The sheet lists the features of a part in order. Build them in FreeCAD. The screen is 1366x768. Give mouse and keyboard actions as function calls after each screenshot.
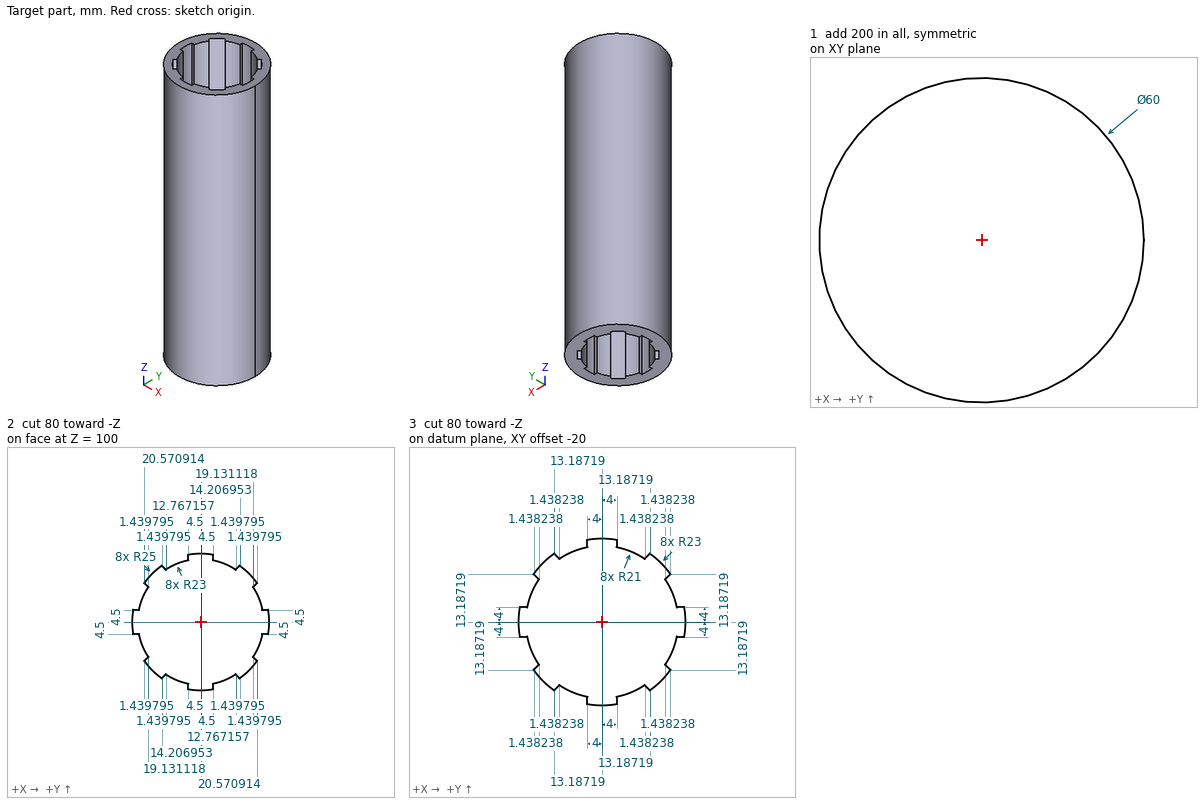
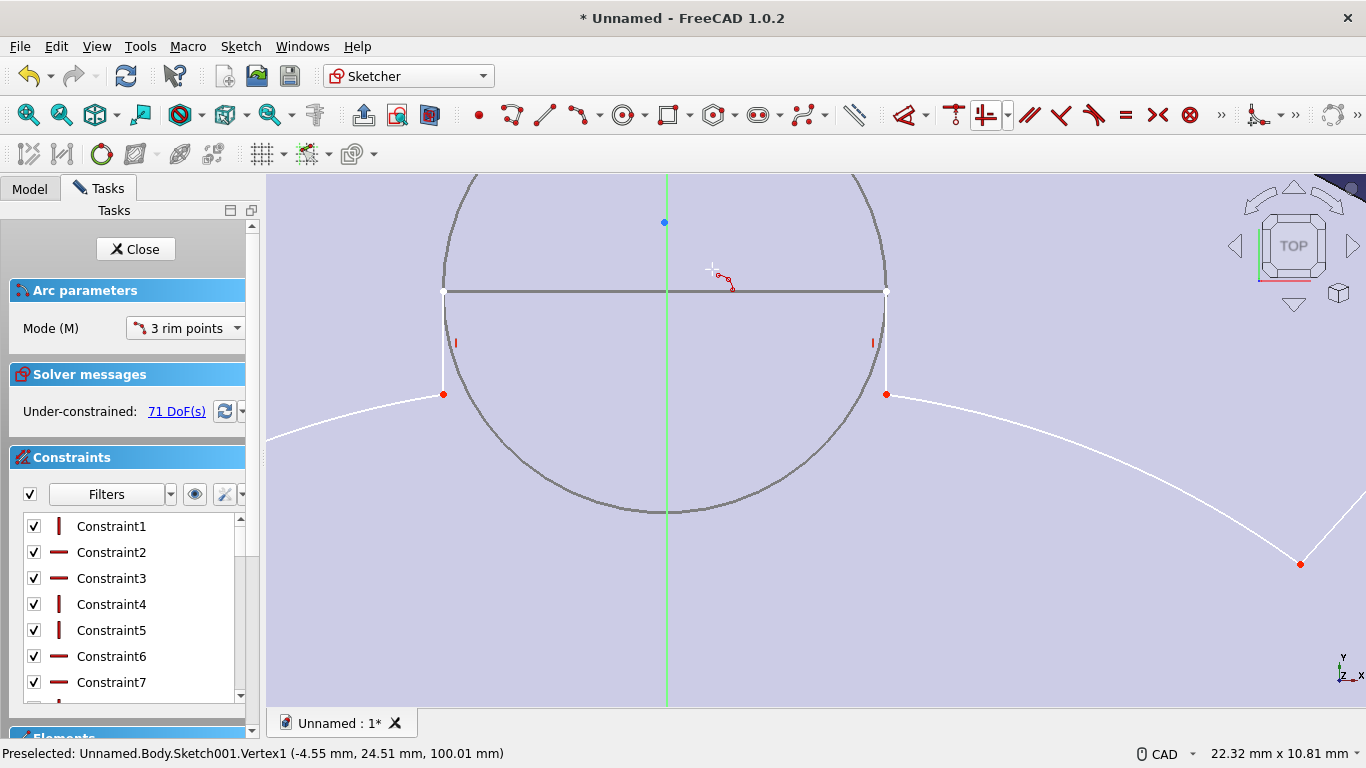
click(712, 268)
key(Escape)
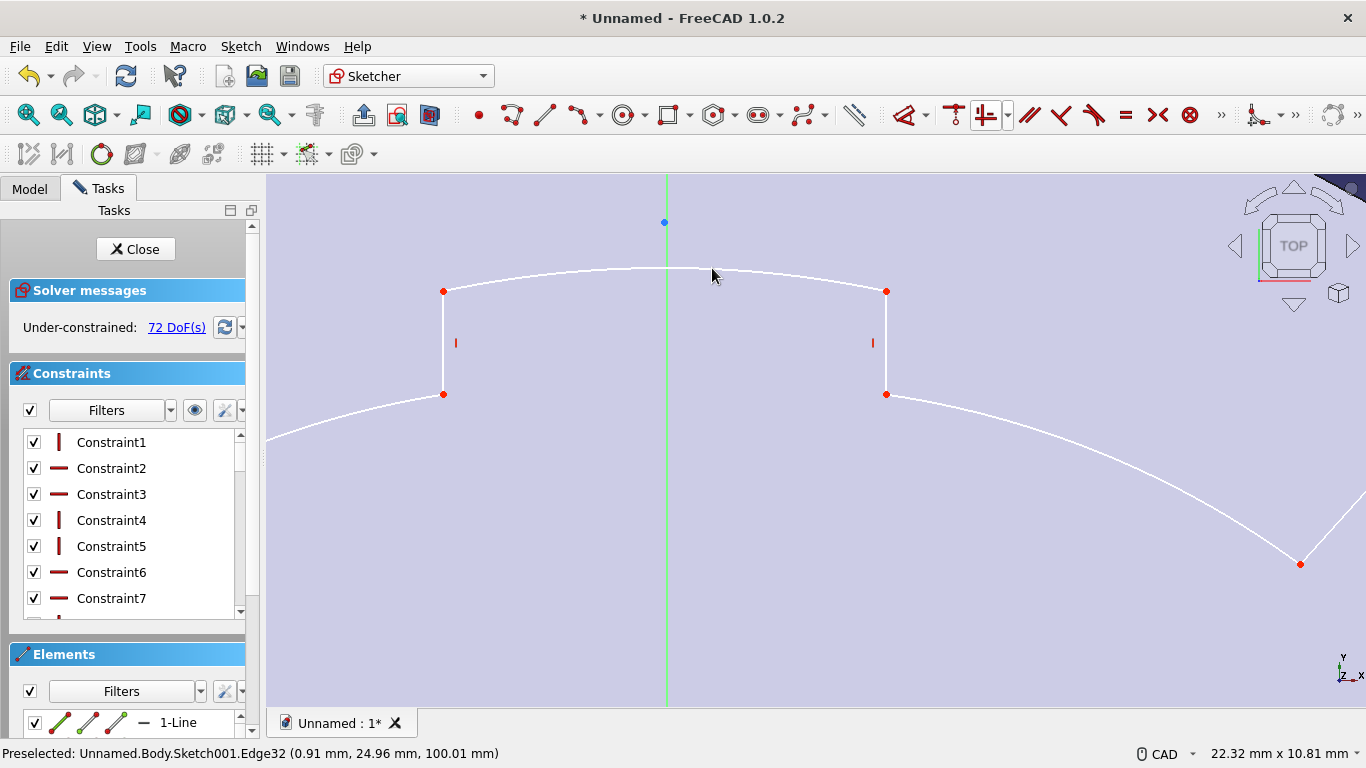
scroll(760, 275, down, 10)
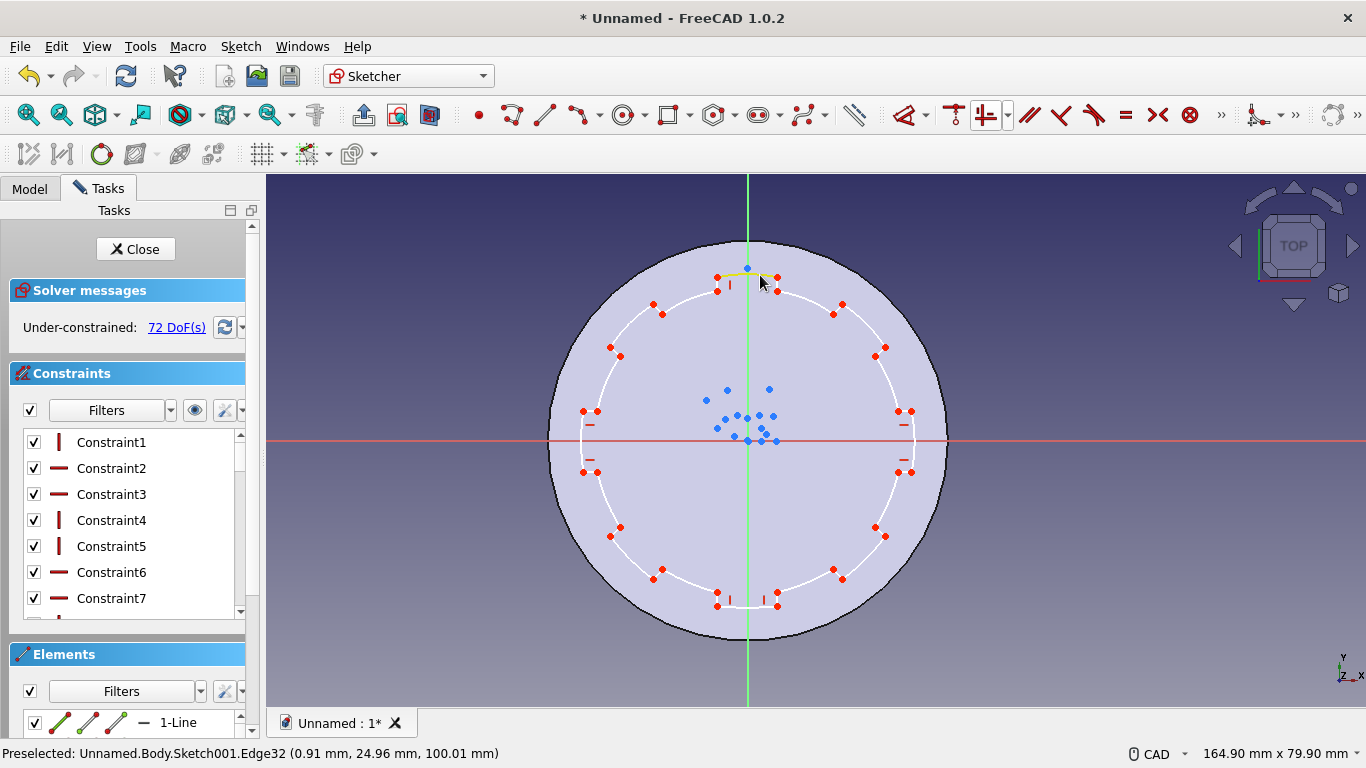
click(700, 295)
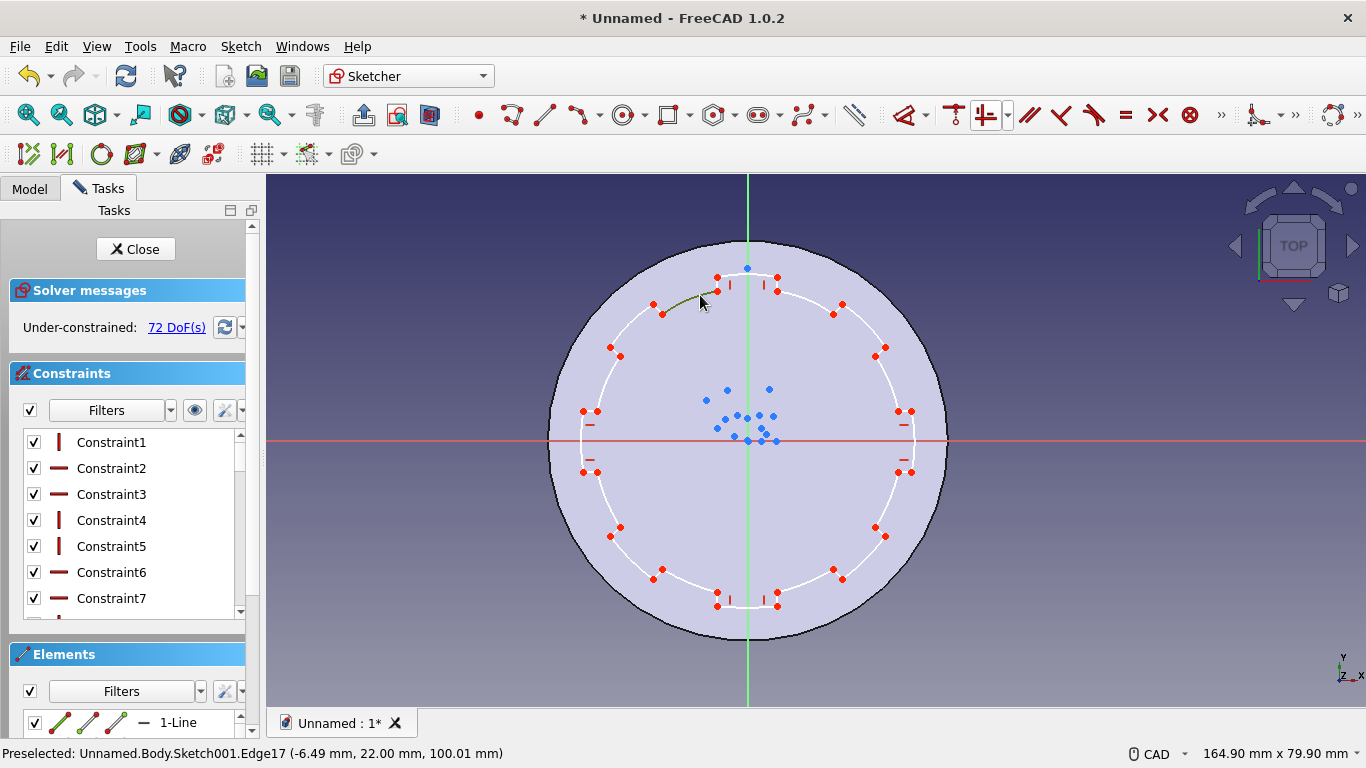
click(639, 315)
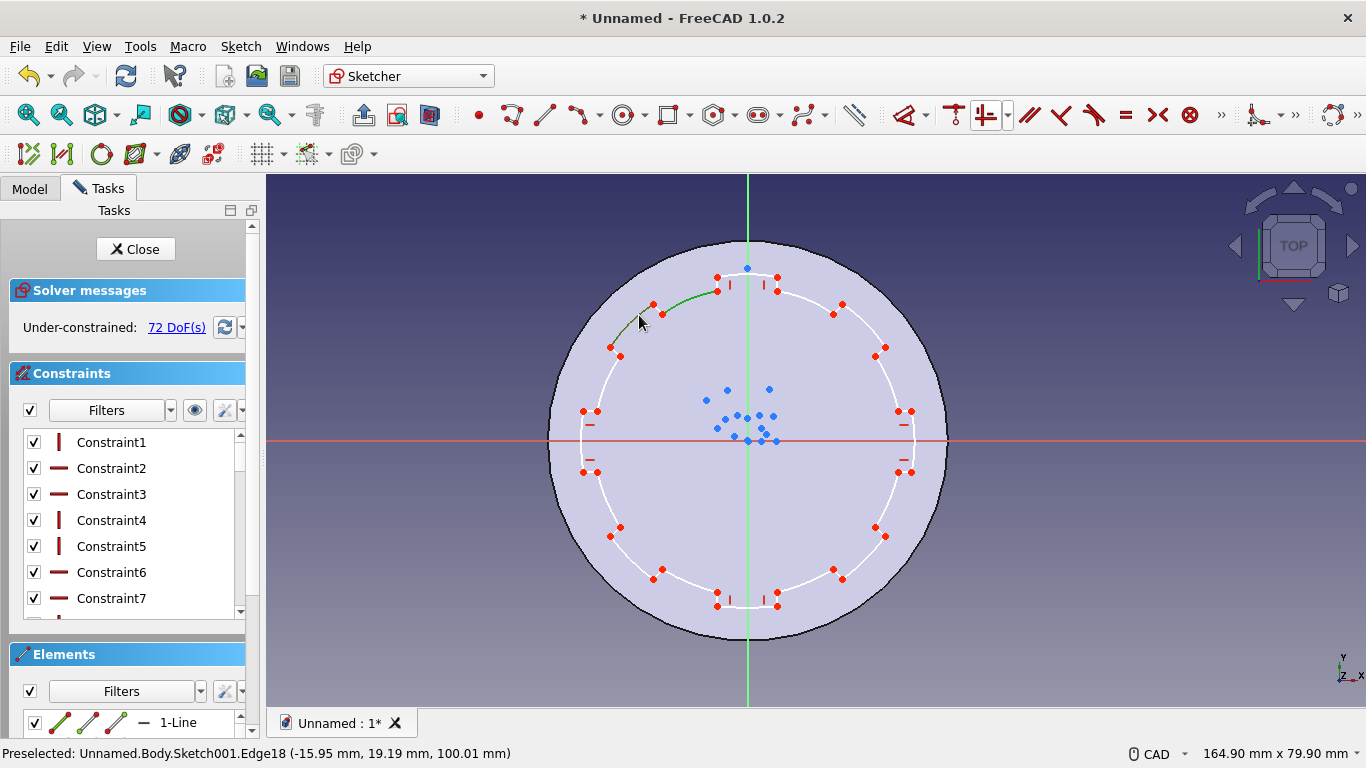
click(954, 116)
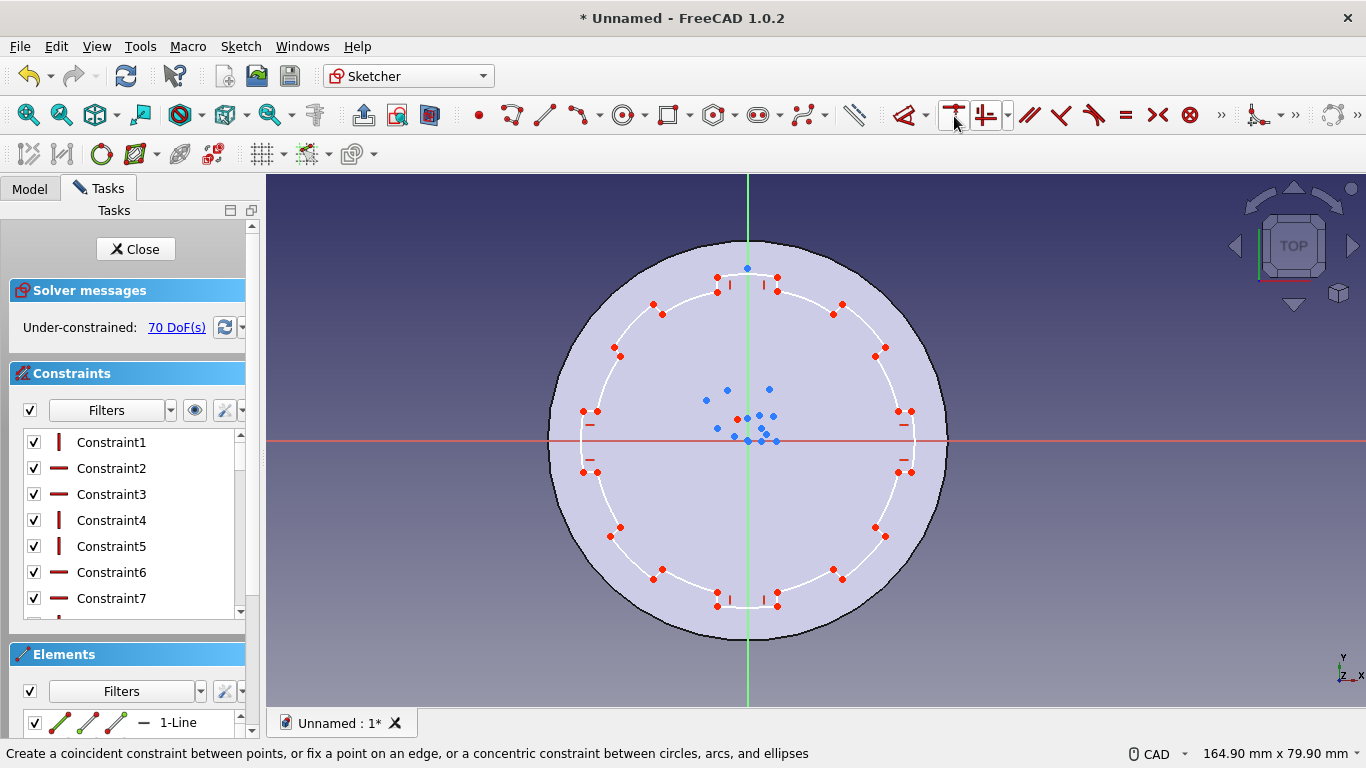
click(700, 296)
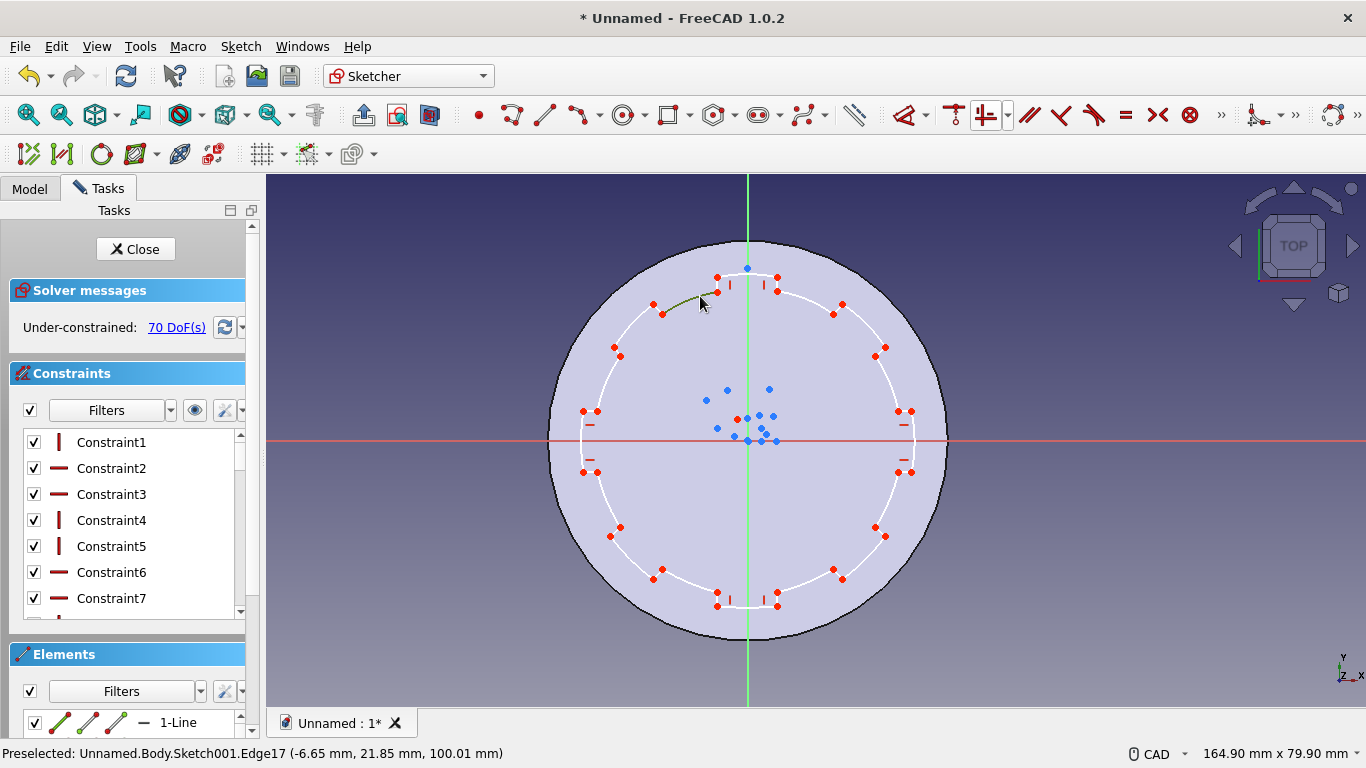
click(611, 372)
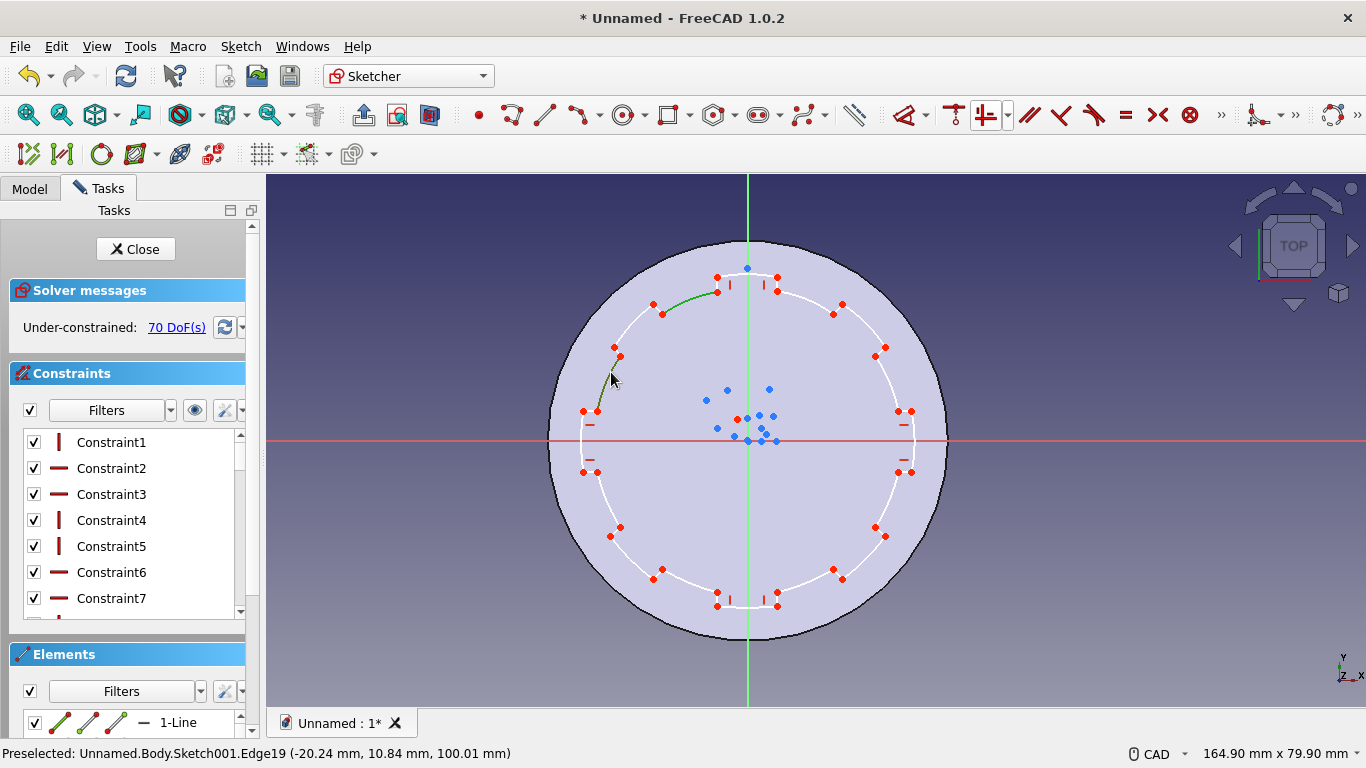
click(954, 116)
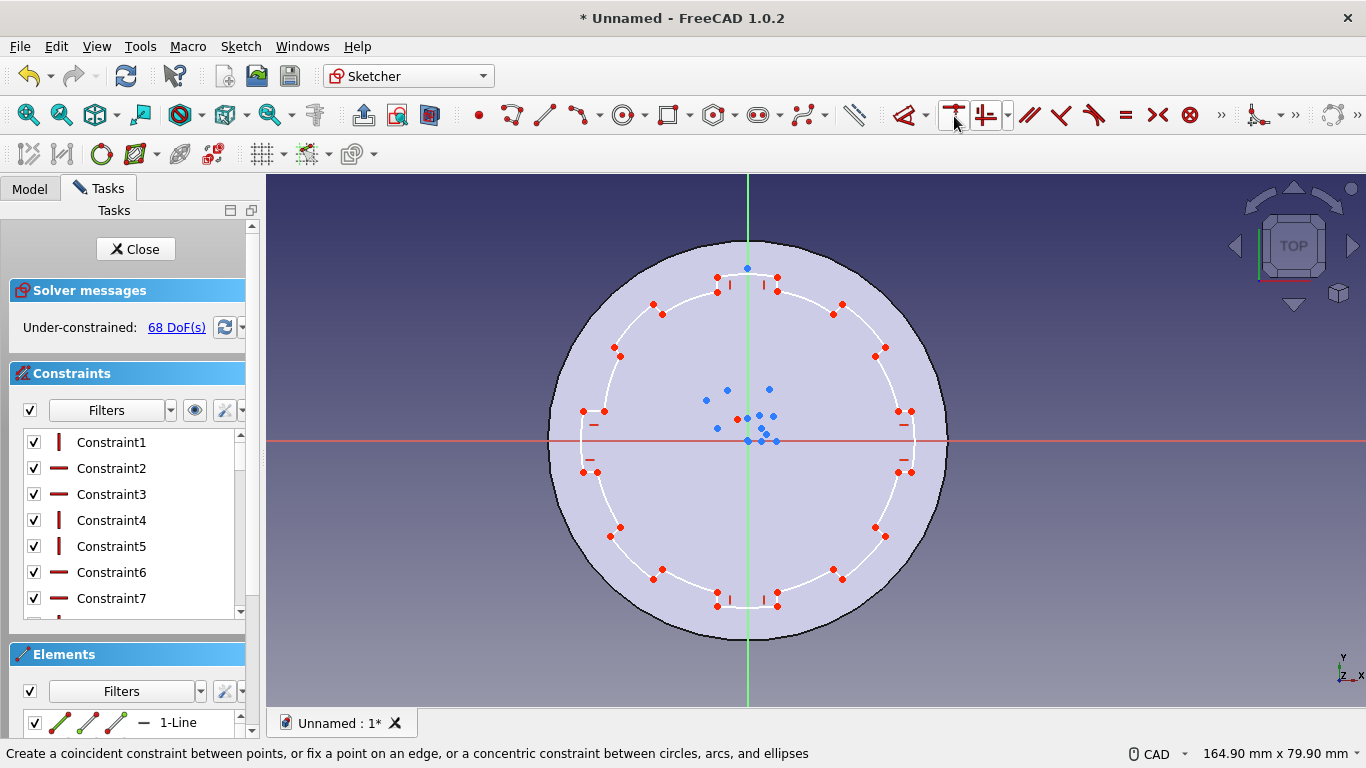
click(700, 296)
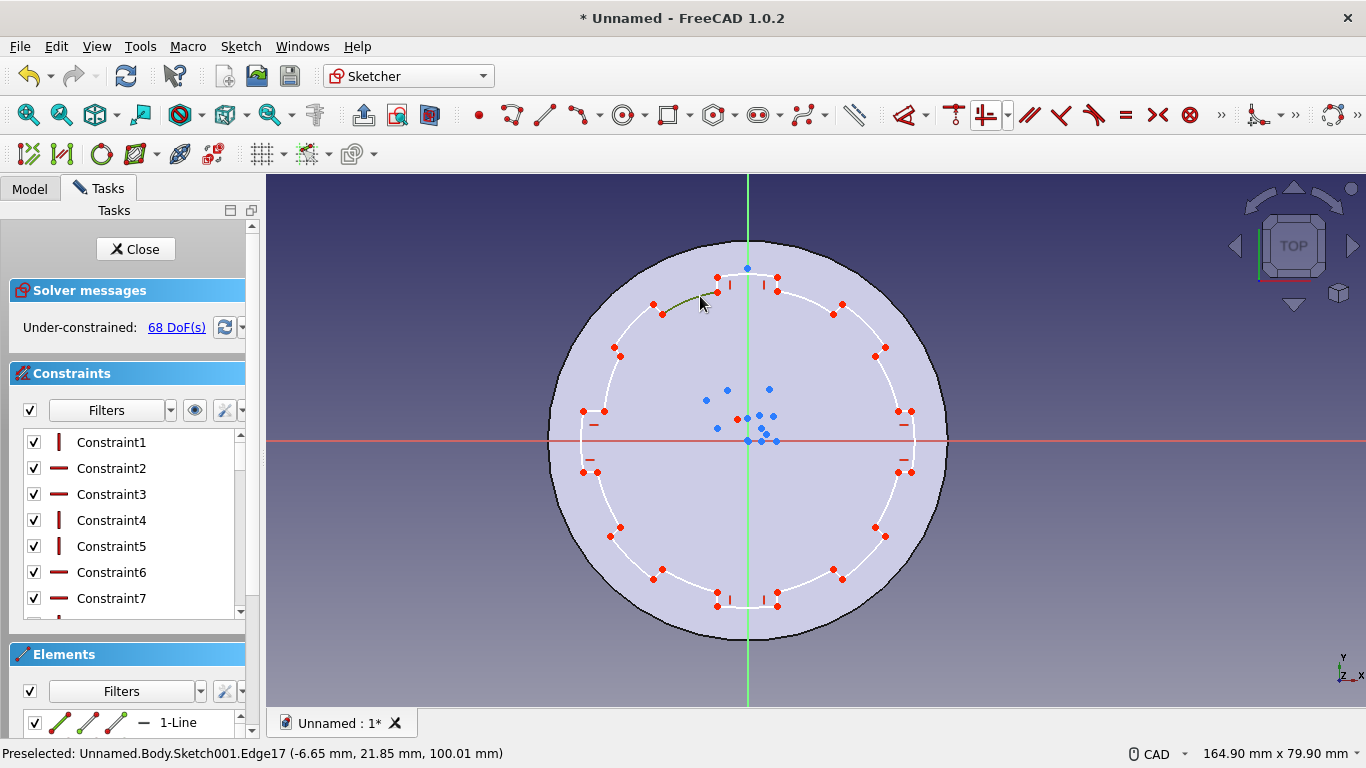
scroll(581, 430, up, 2)